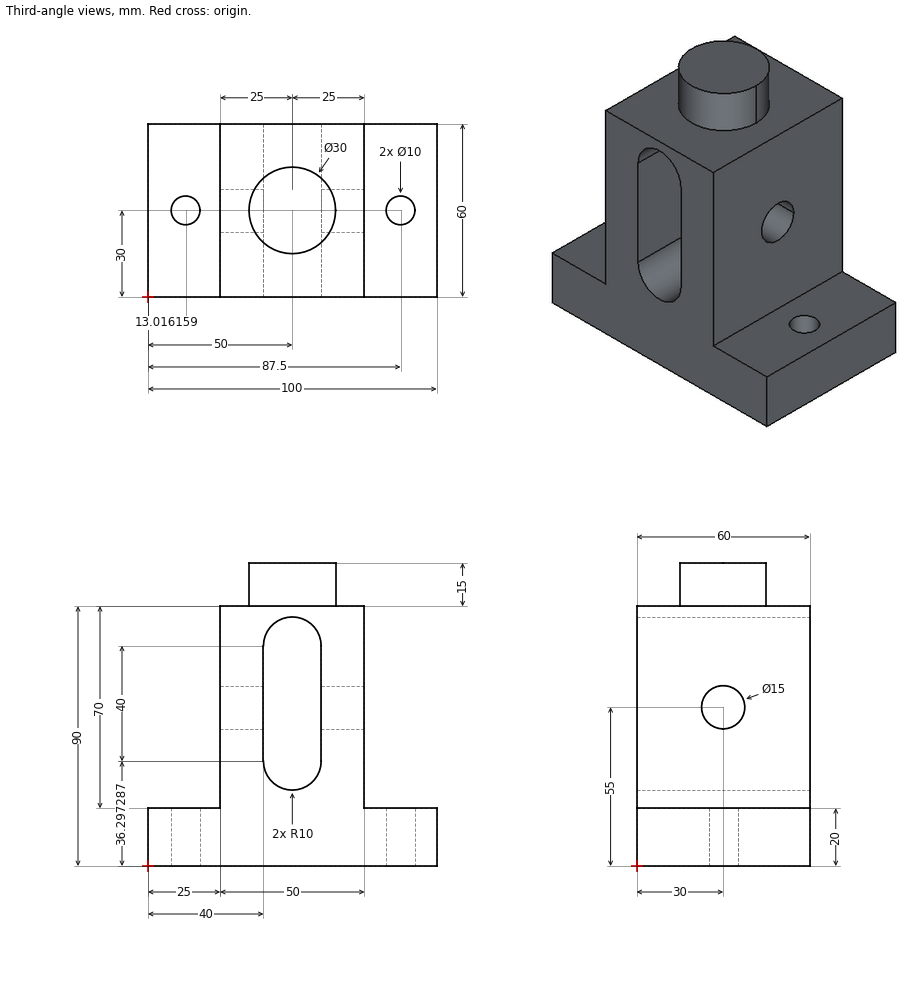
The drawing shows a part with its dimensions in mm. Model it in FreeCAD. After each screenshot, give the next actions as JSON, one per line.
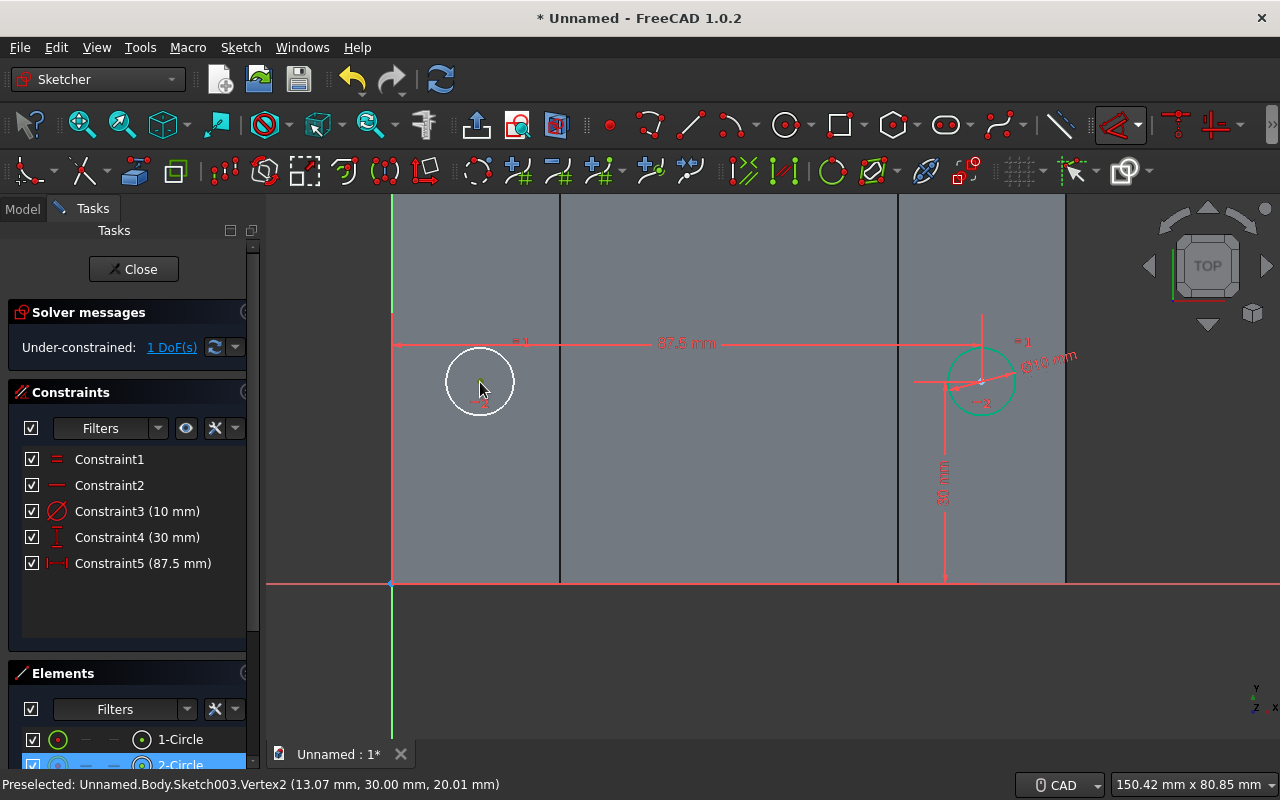
{"action": "key", "text": "l"}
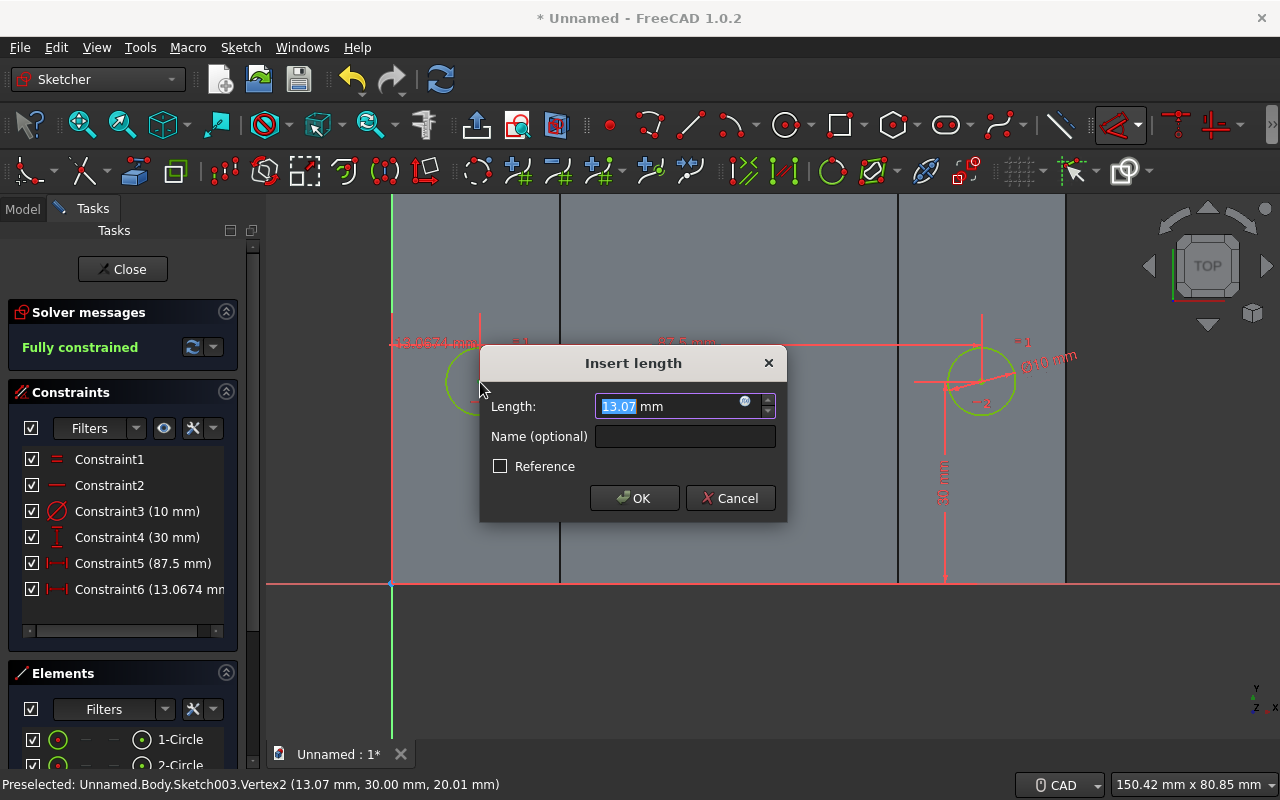
{"action": "type", "text": "13.016159"}
{"action": "key", "text": "Return"}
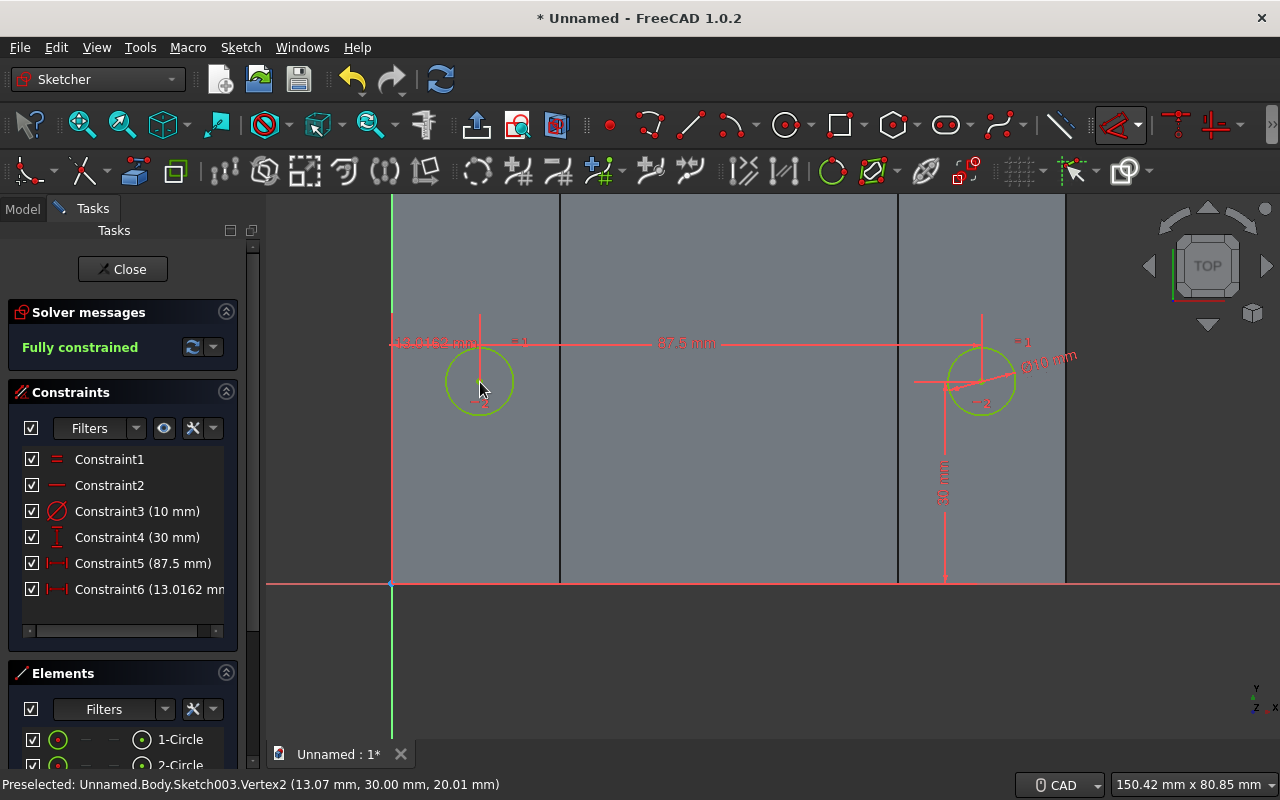
{"action": "left_click", "coordinate": [123, 269]}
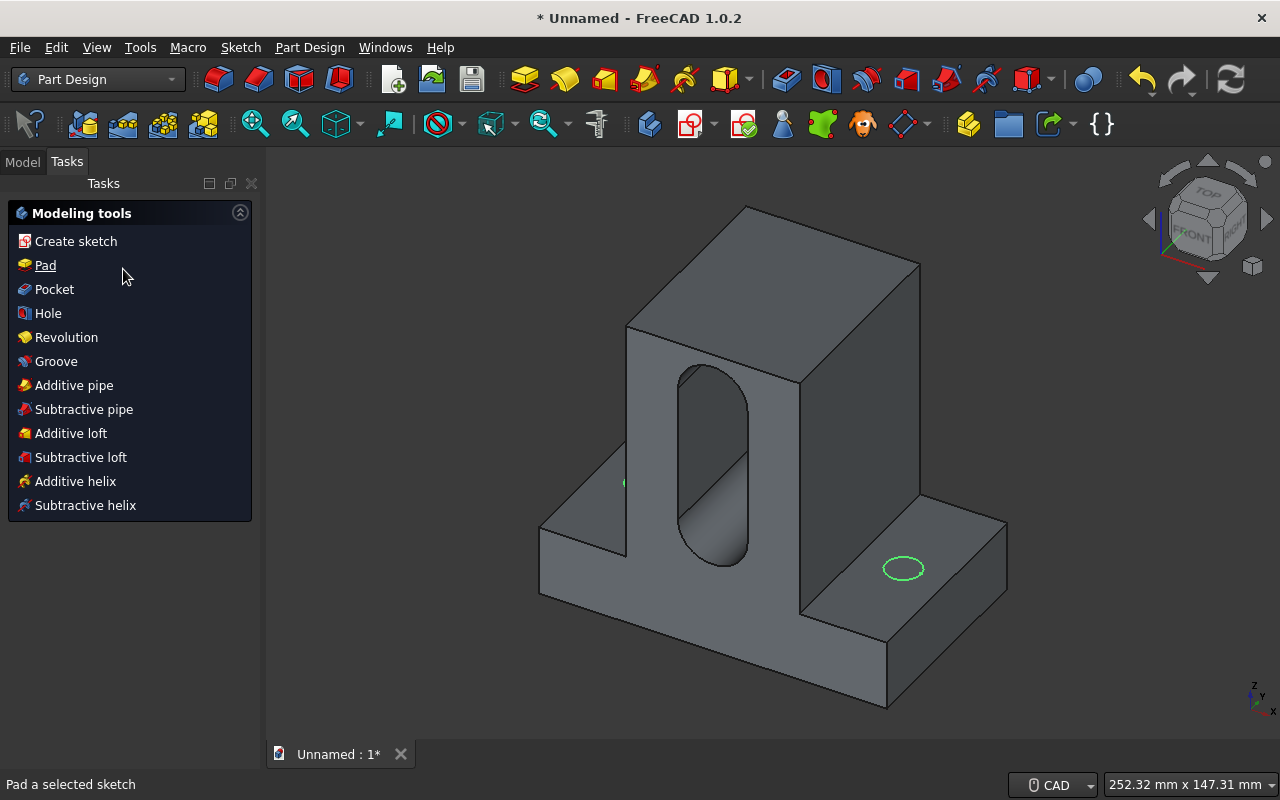
{"action": "left_click", "coordinate": [788, 80]}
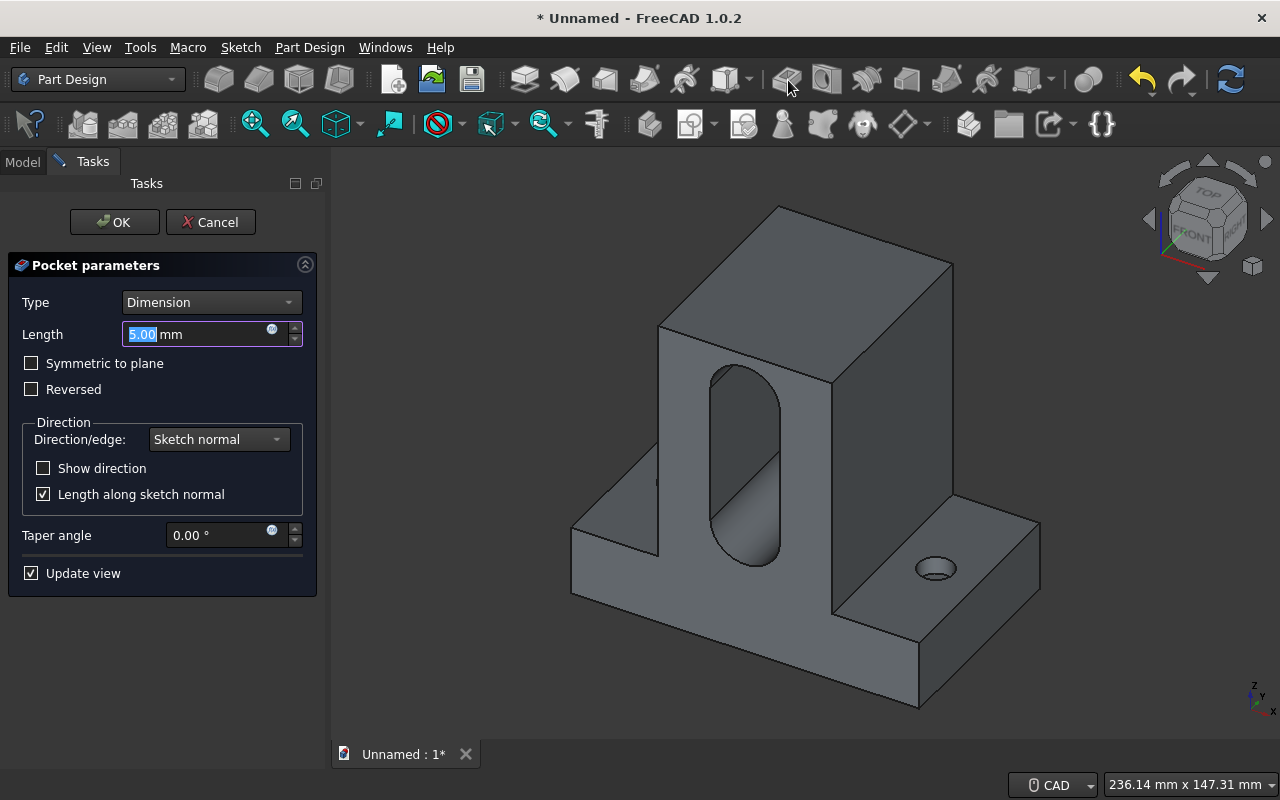
{"action": "type", "text": "20"}
{"action": "key", "text": "Tab"}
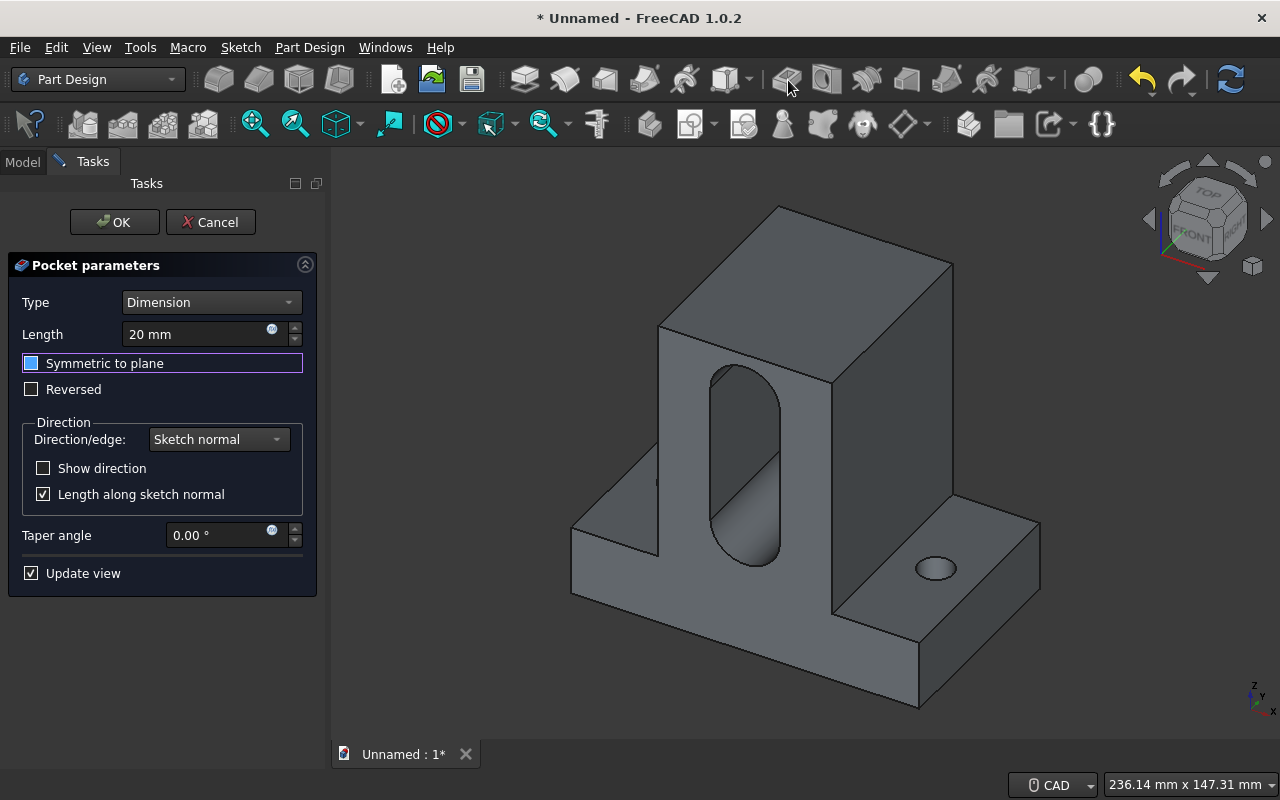
{"action": "left_click", "coordinate": [115, 222]}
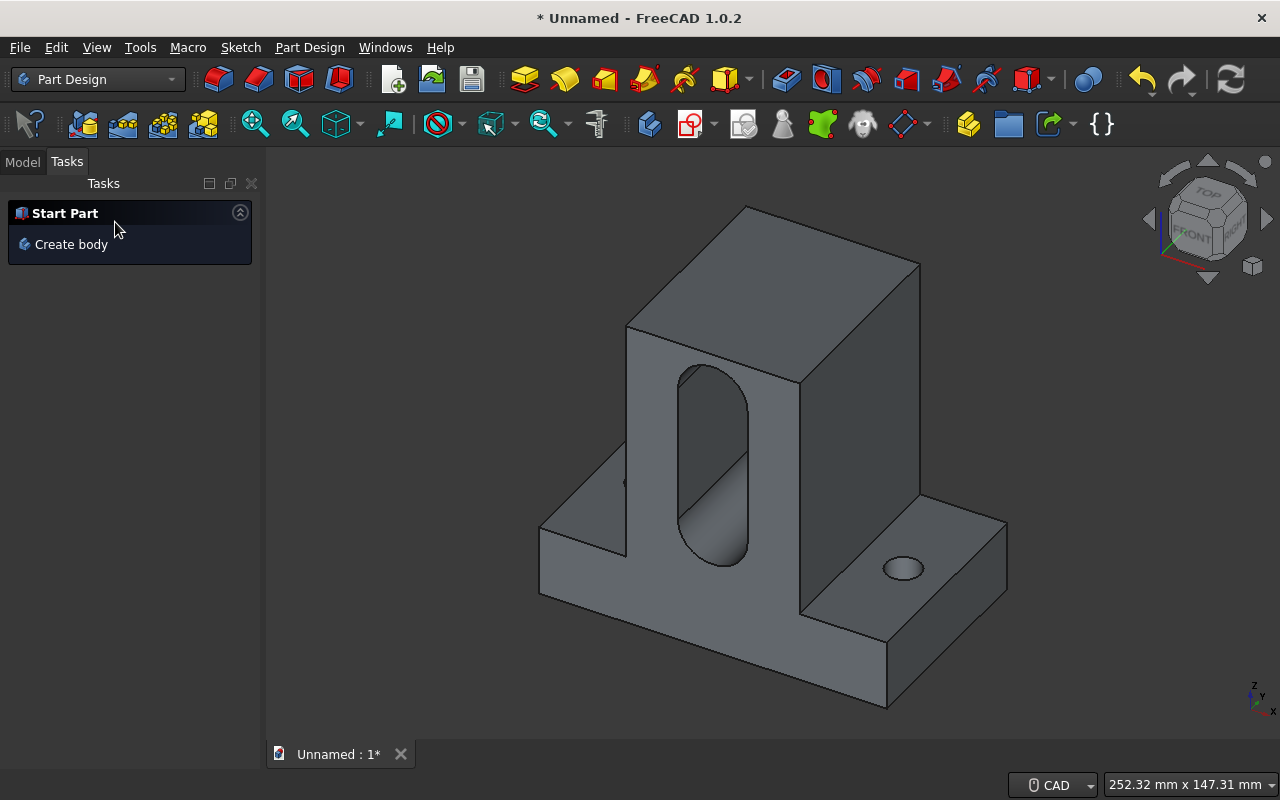
{"action": "left_click", "coordinate": [860, 438]}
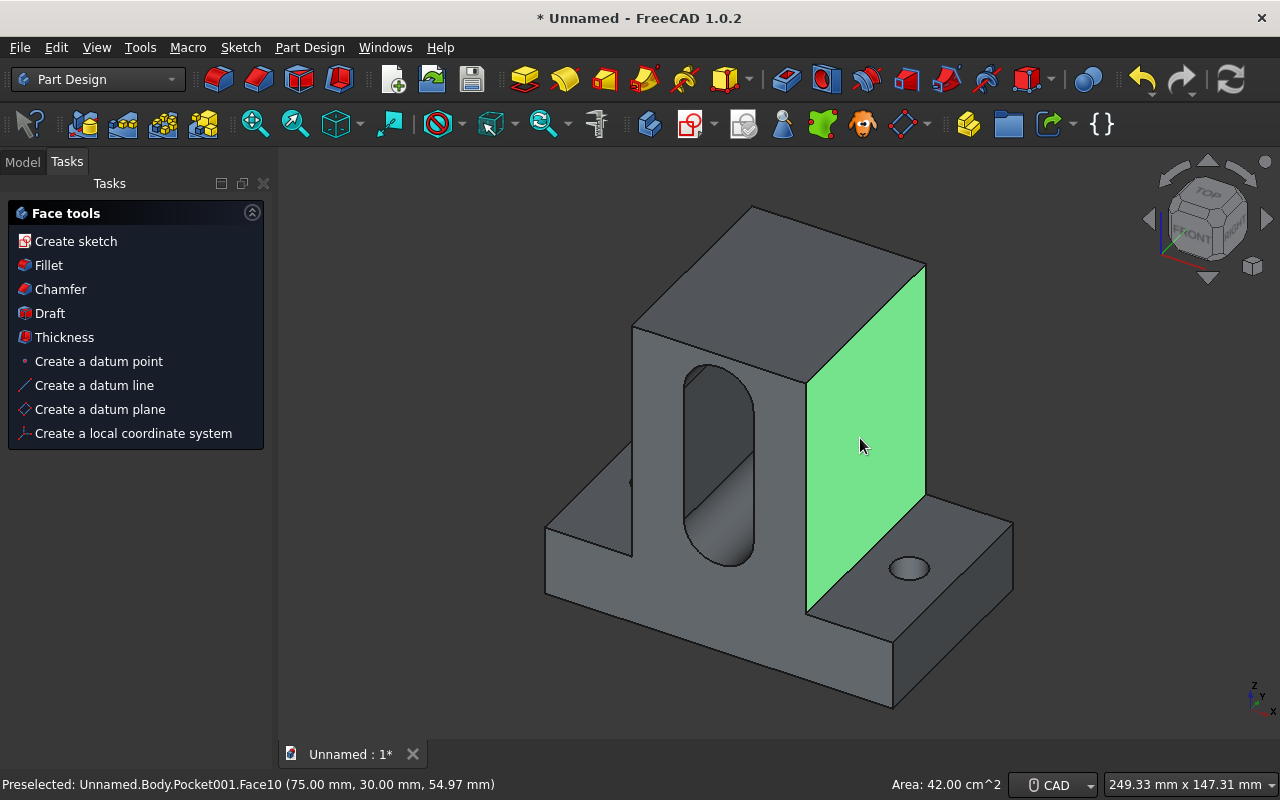
{"action": "left_click", "coordinate": [690, 124]}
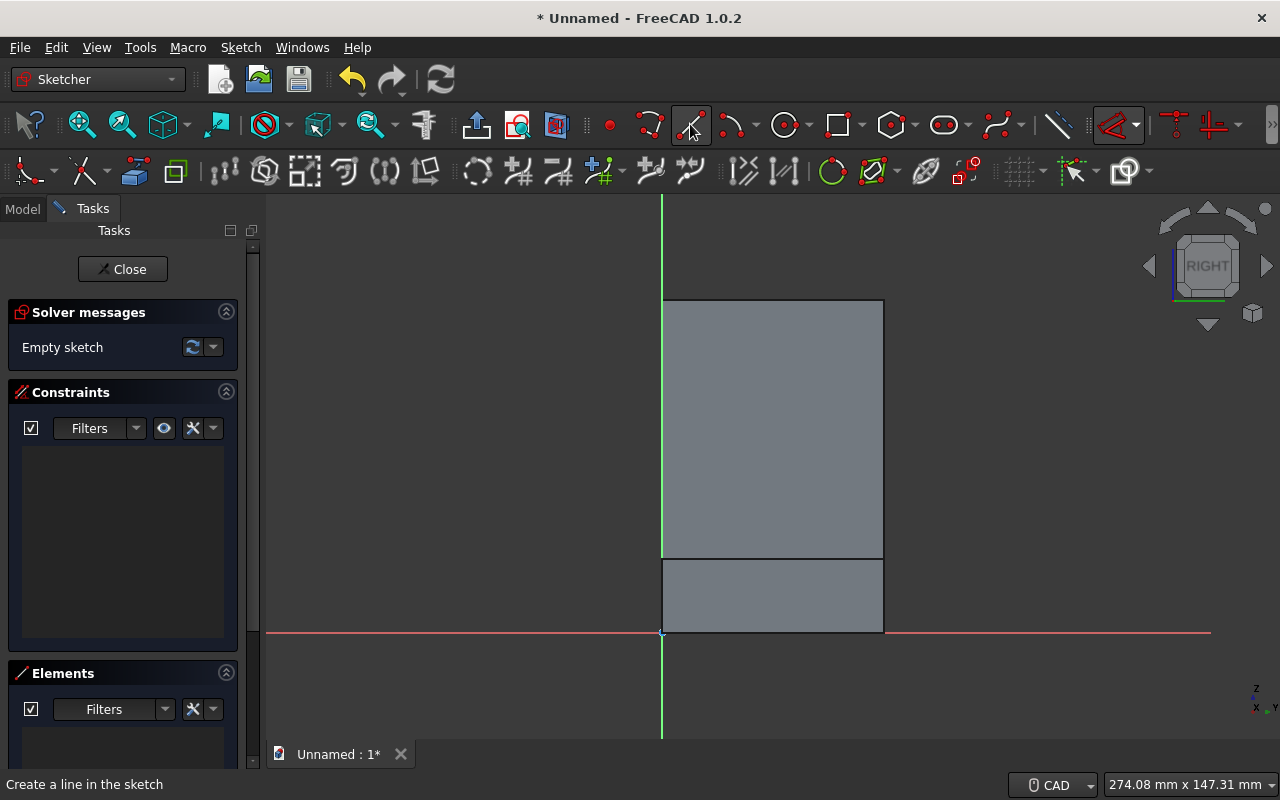
{"action": "left_click", "coordinate": [558, 126]}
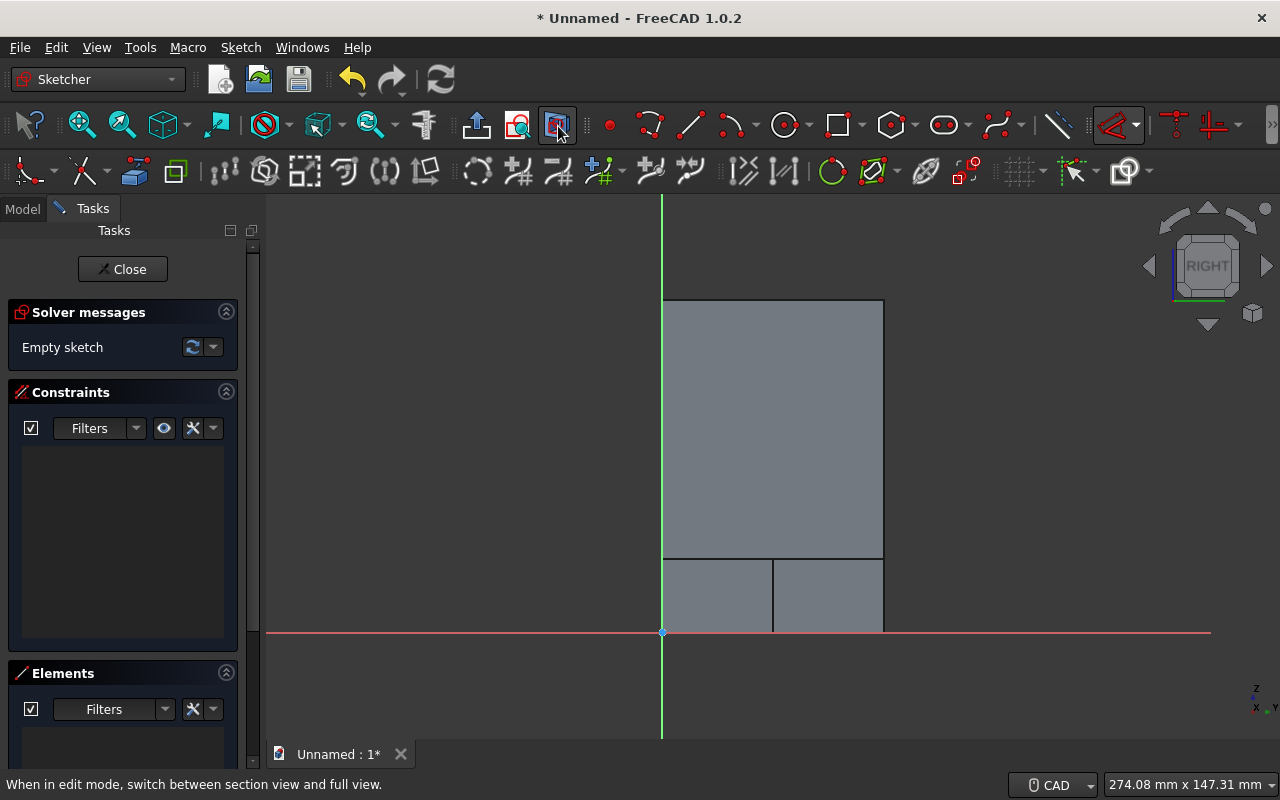
{"action": "scroll", "coordinate": [787, 422], "scroll_direction": "up", "scroll_amount": 9}